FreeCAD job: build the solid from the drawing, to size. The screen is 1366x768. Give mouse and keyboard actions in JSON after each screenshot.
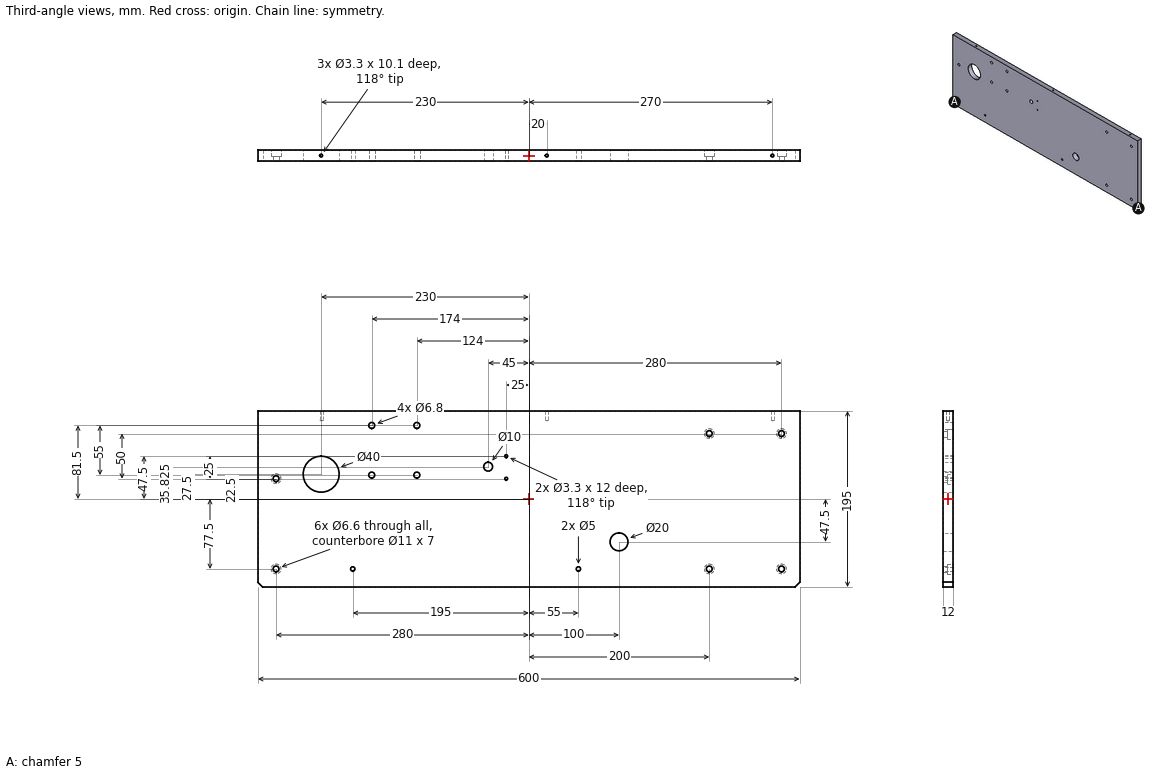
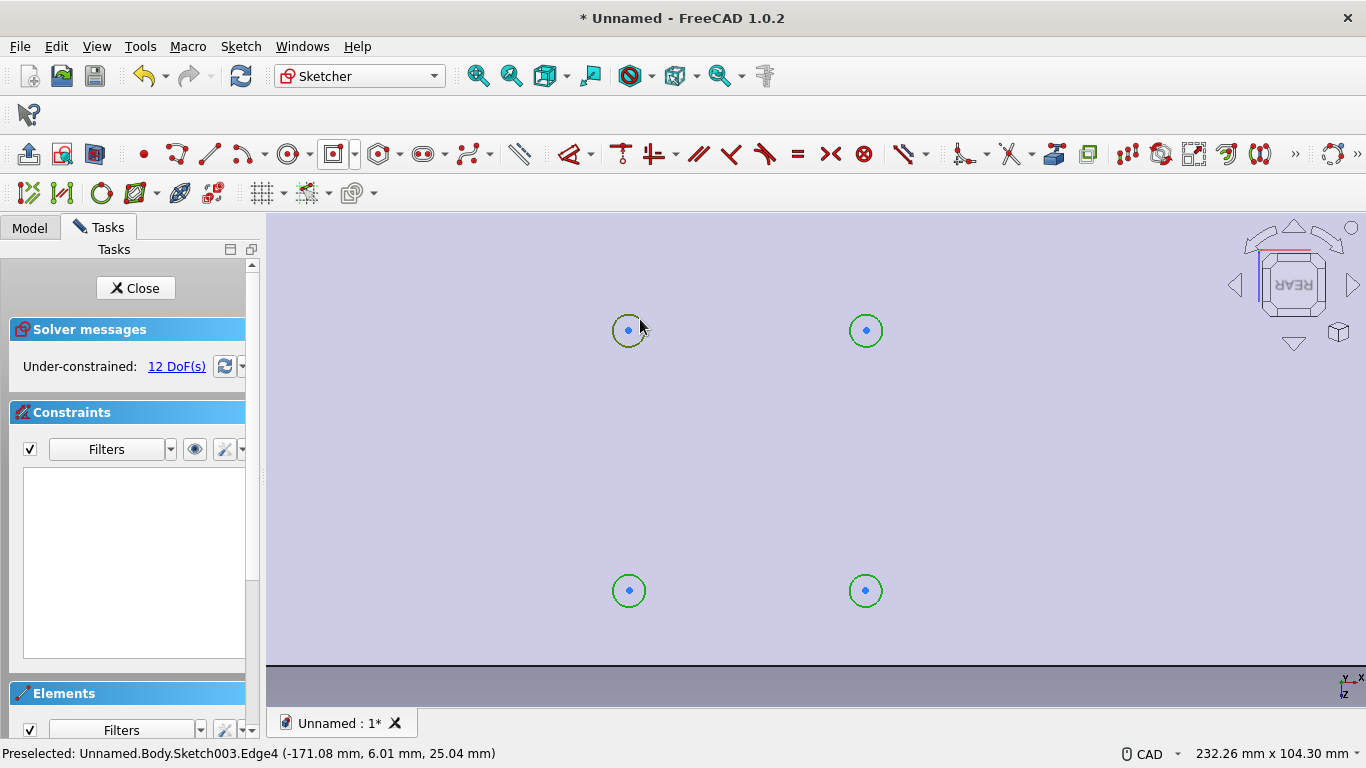
{"action": "left_click", "coordinate": [798, 154]}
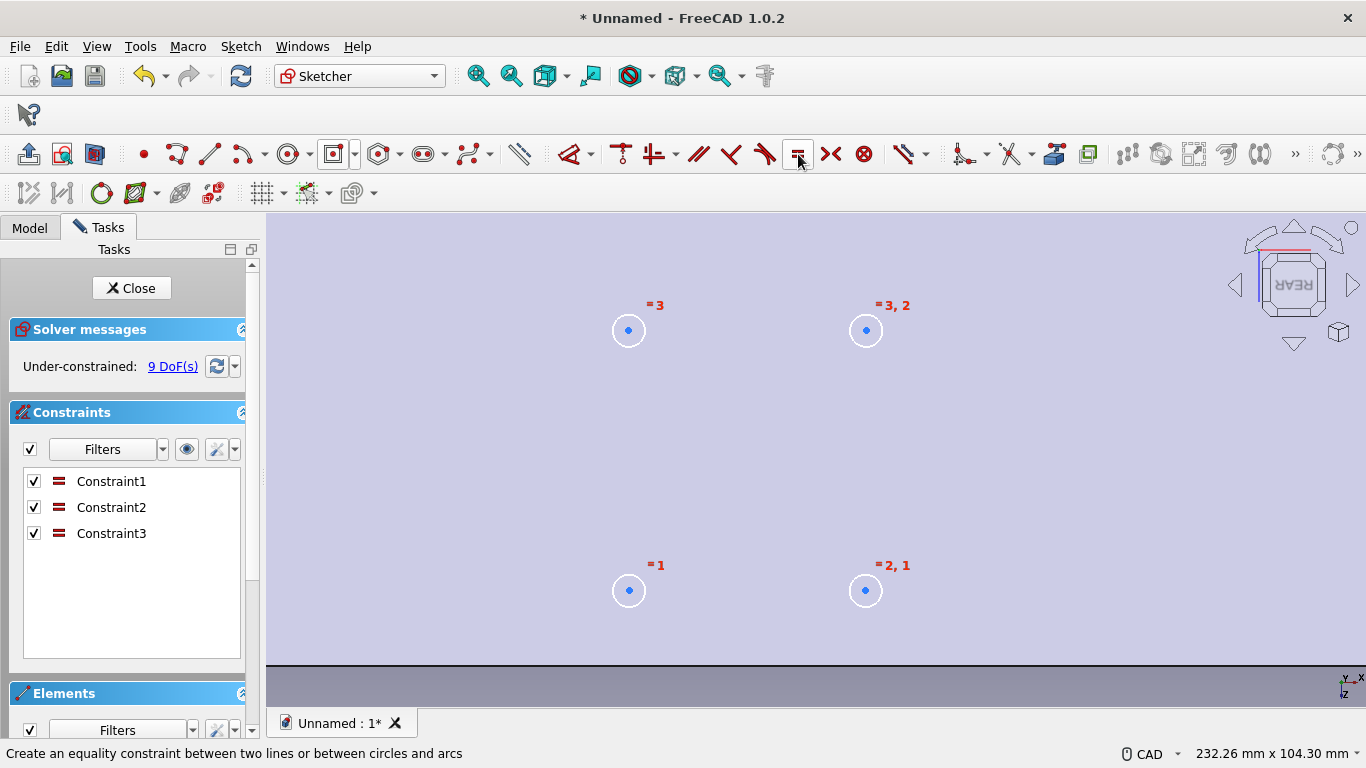
{"action": "key", "text": "d"}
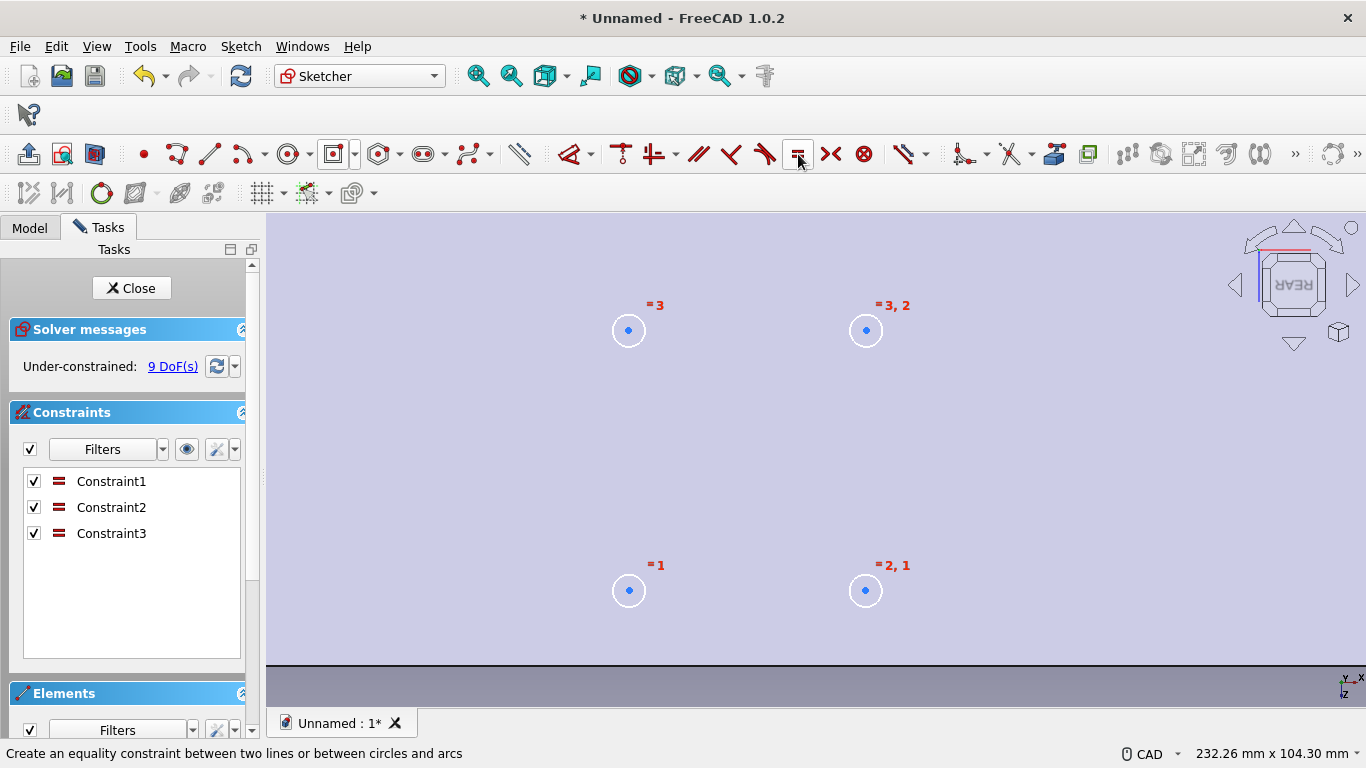
{"action": "scroll", "coordinate": [640, 579], "scroll_direction": "up", "scroll_amount": 2}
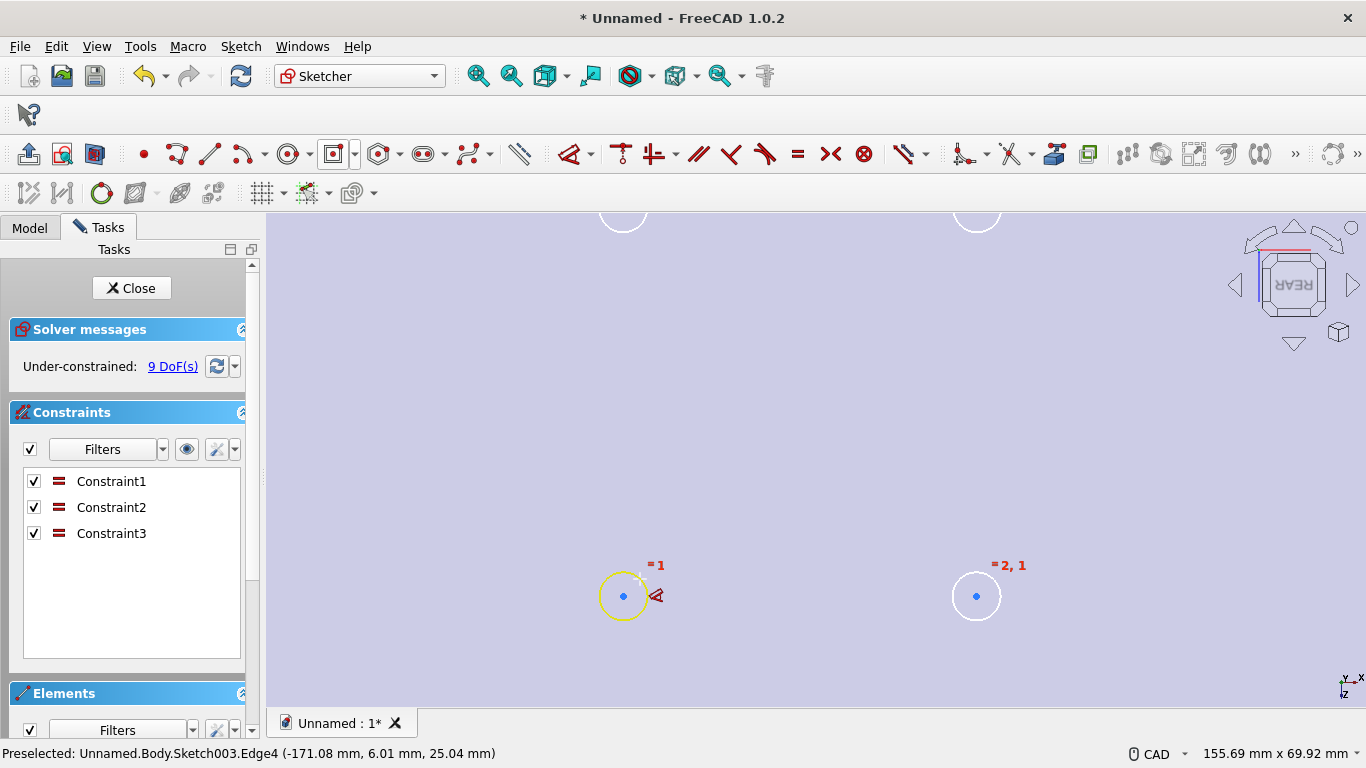
{"action": "left_click", "coordinate": [640, 579]}
{"action": "left_click", "coordinate": [662, 556]}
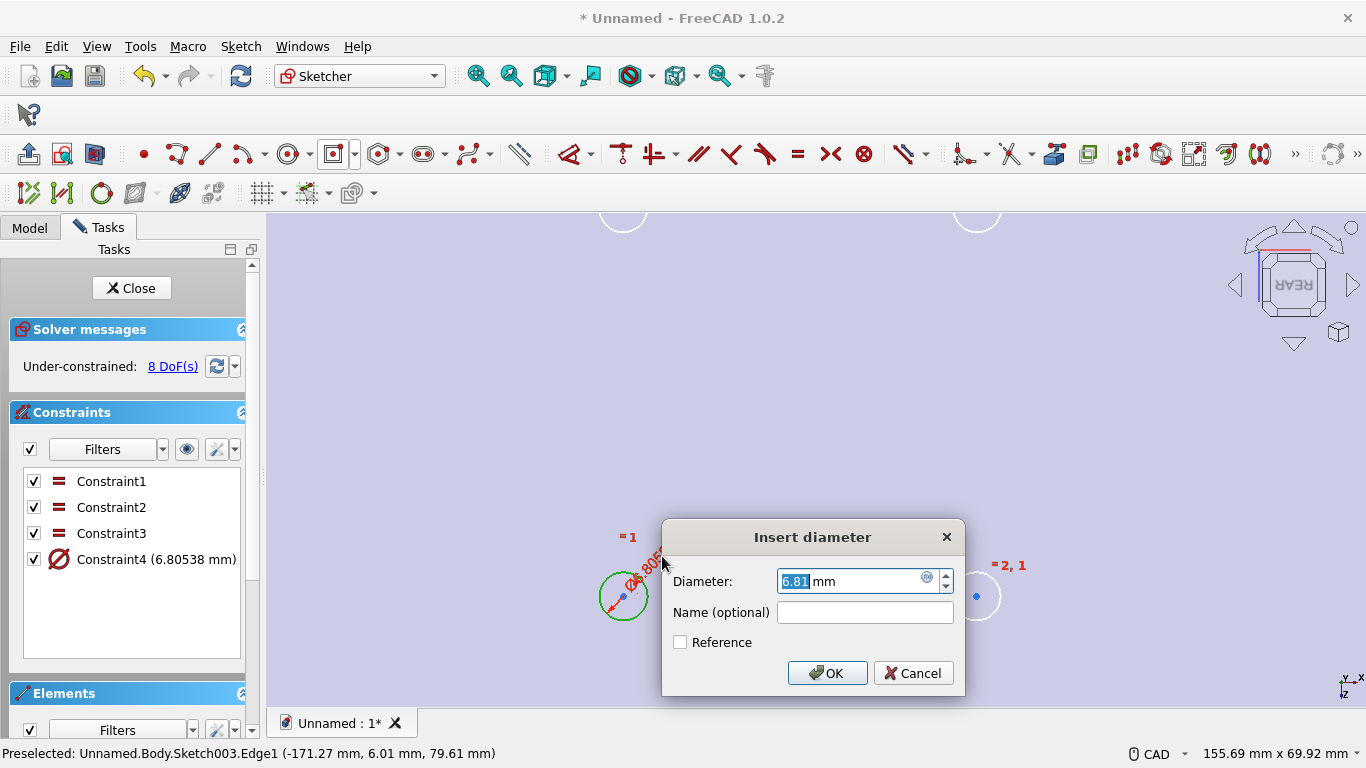
{"action": "type", "text": "6.8"}
{"action": "key", "text": "Return"}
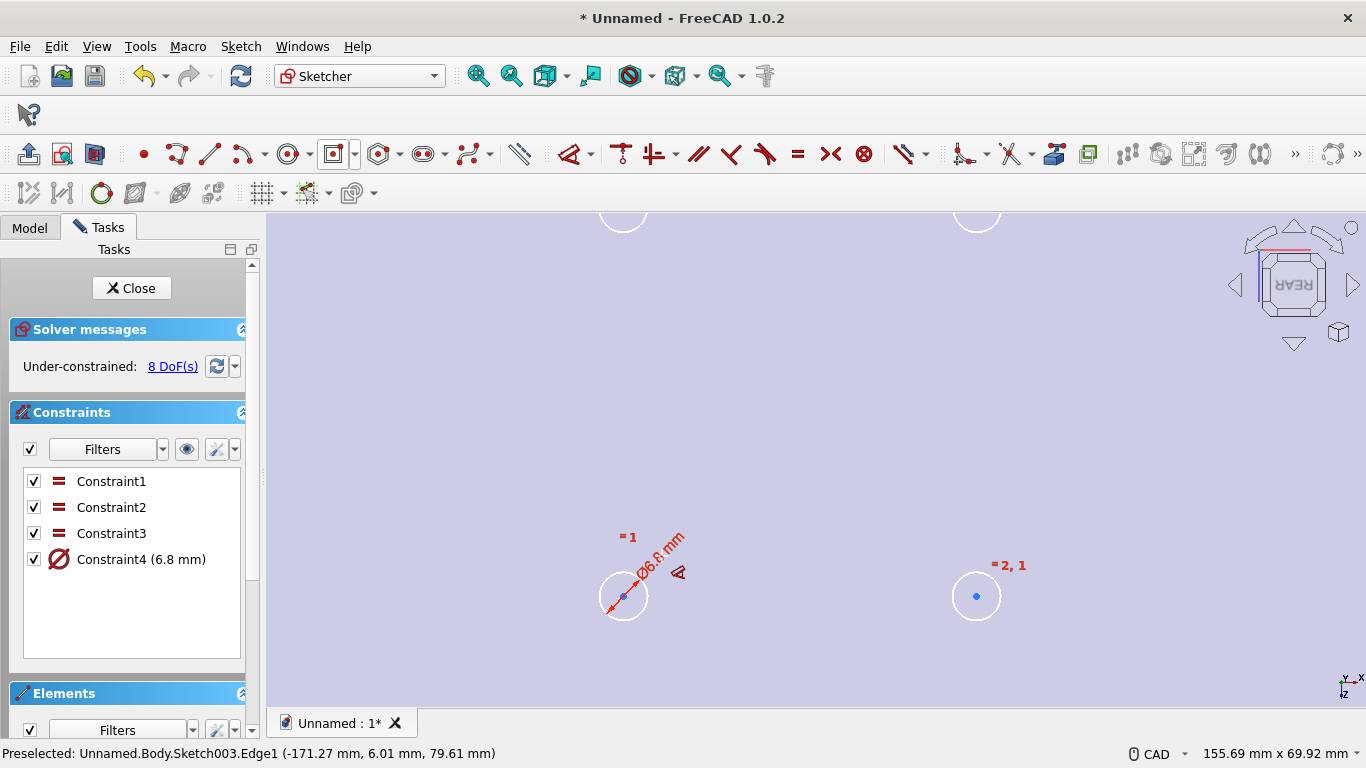
{"action": "left_click", "coordinate": [624, 596]}
{"action": "left_click", "coordinate": [912, 630]}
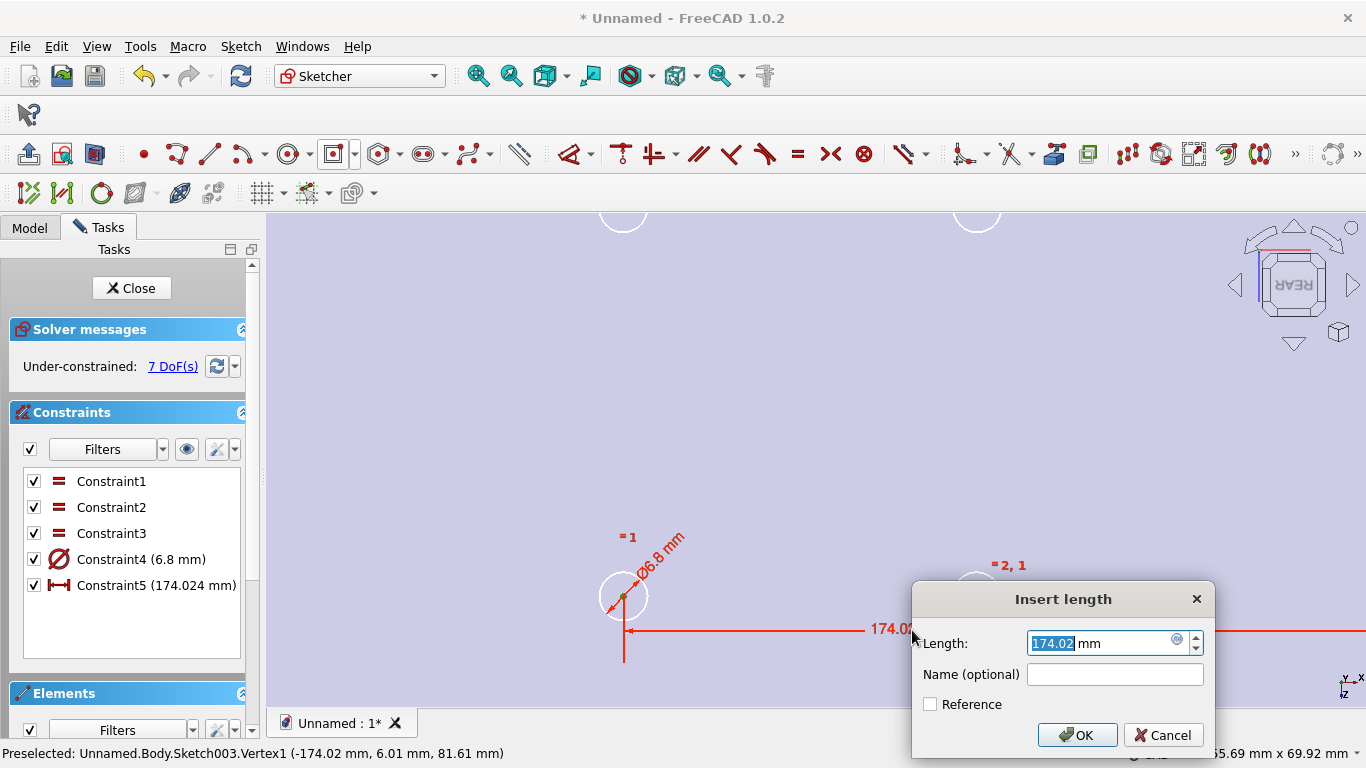
{"action": "type", "text": "174"}
{"action": "key", "text": "Return"}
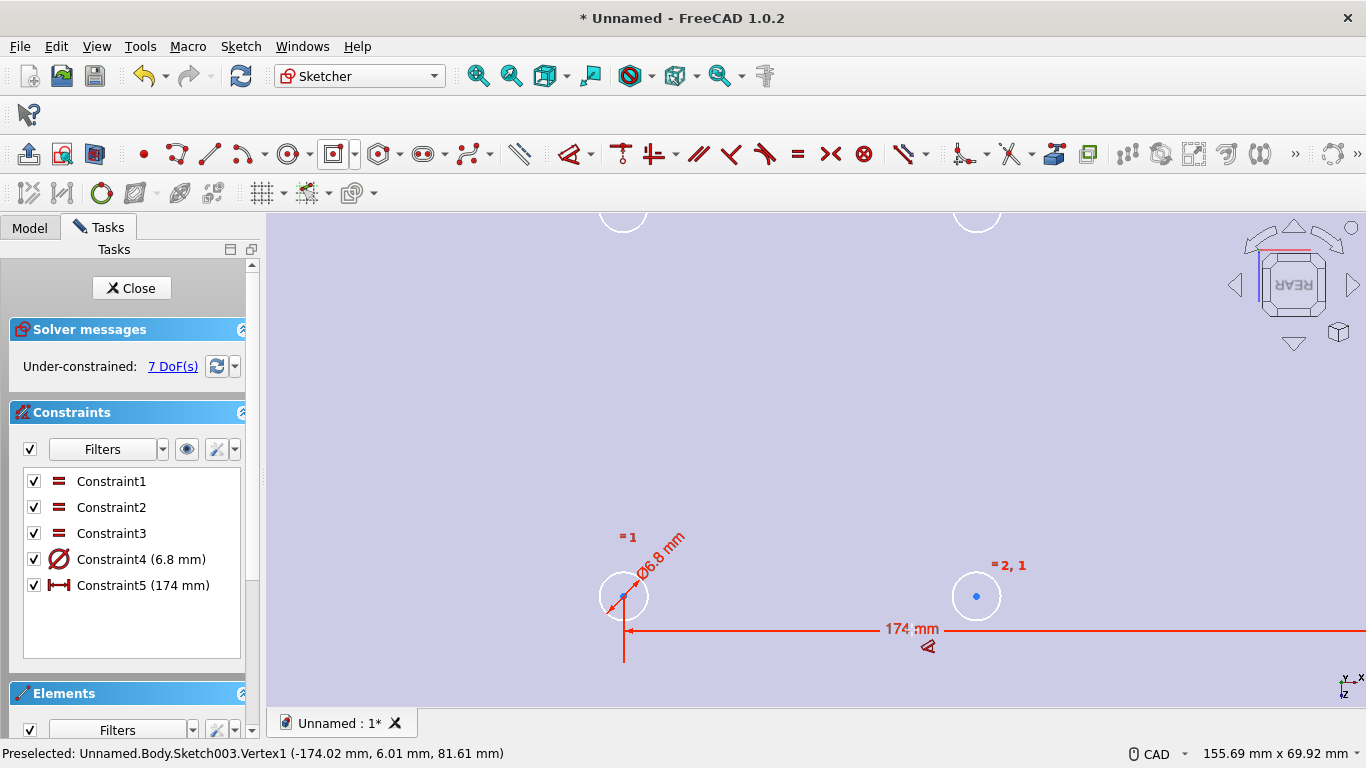
{"action": "left_click", "coordinate": [977, 596]}
{"action": "left_click", "coordinate": [1089, 630]}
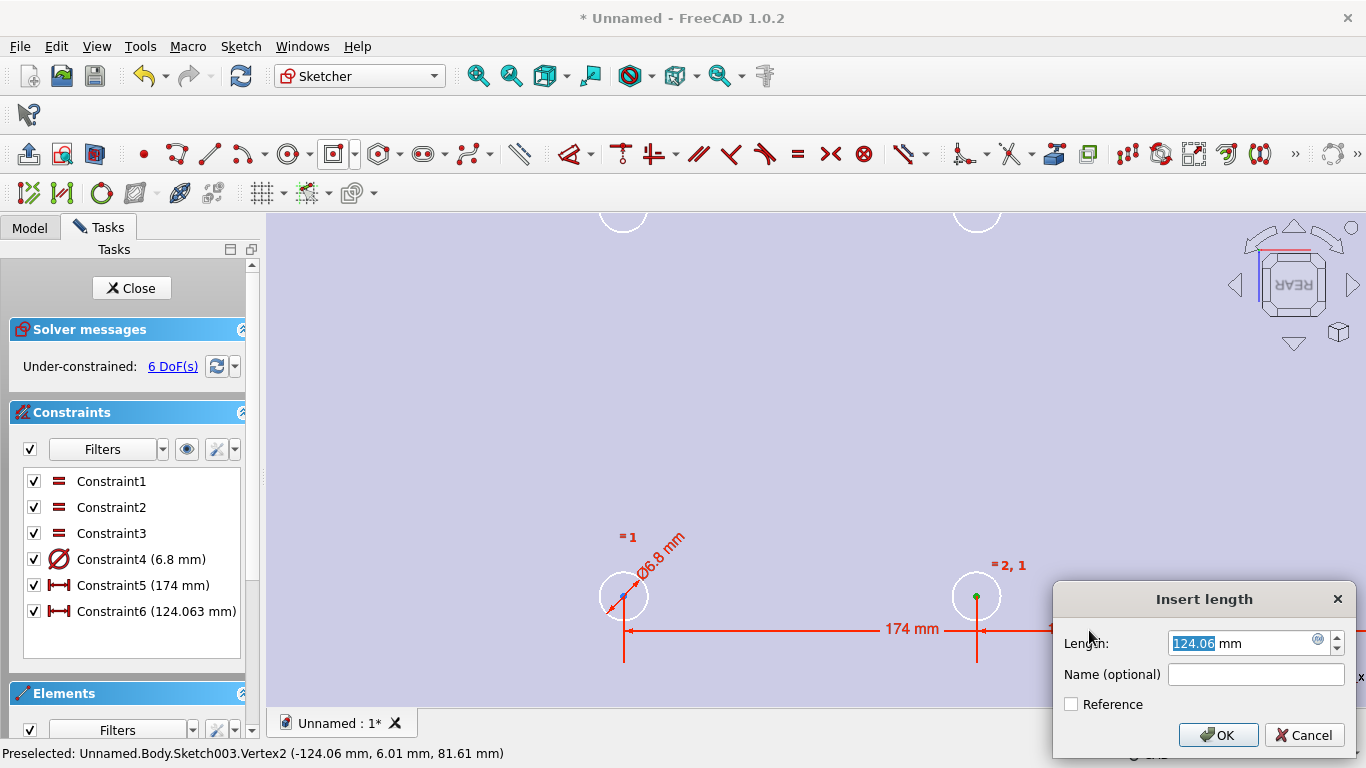
{"action": "type", "text": "124"}
{"action": "key", "text": "Return"}